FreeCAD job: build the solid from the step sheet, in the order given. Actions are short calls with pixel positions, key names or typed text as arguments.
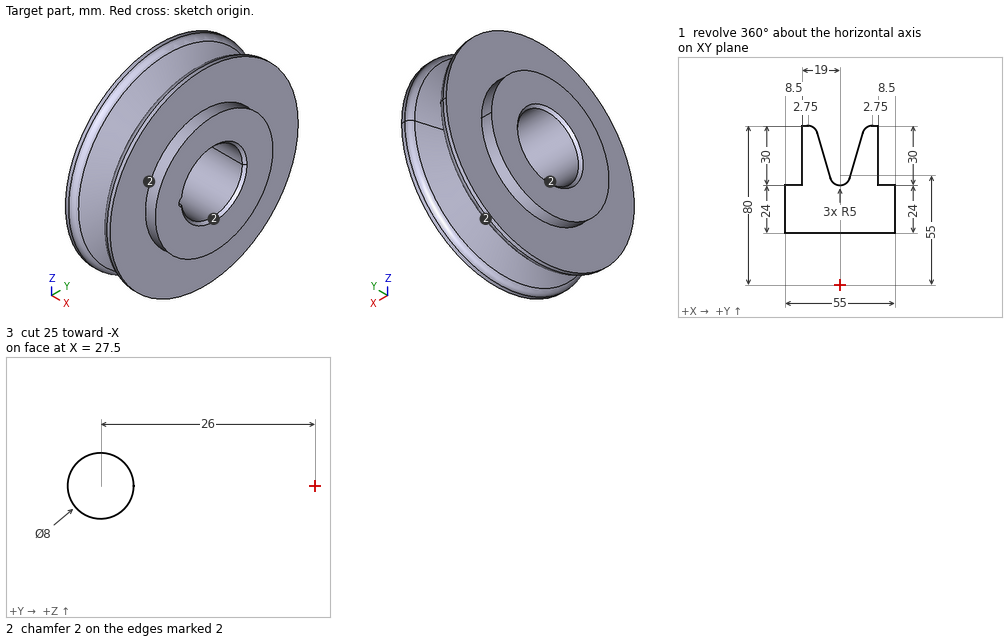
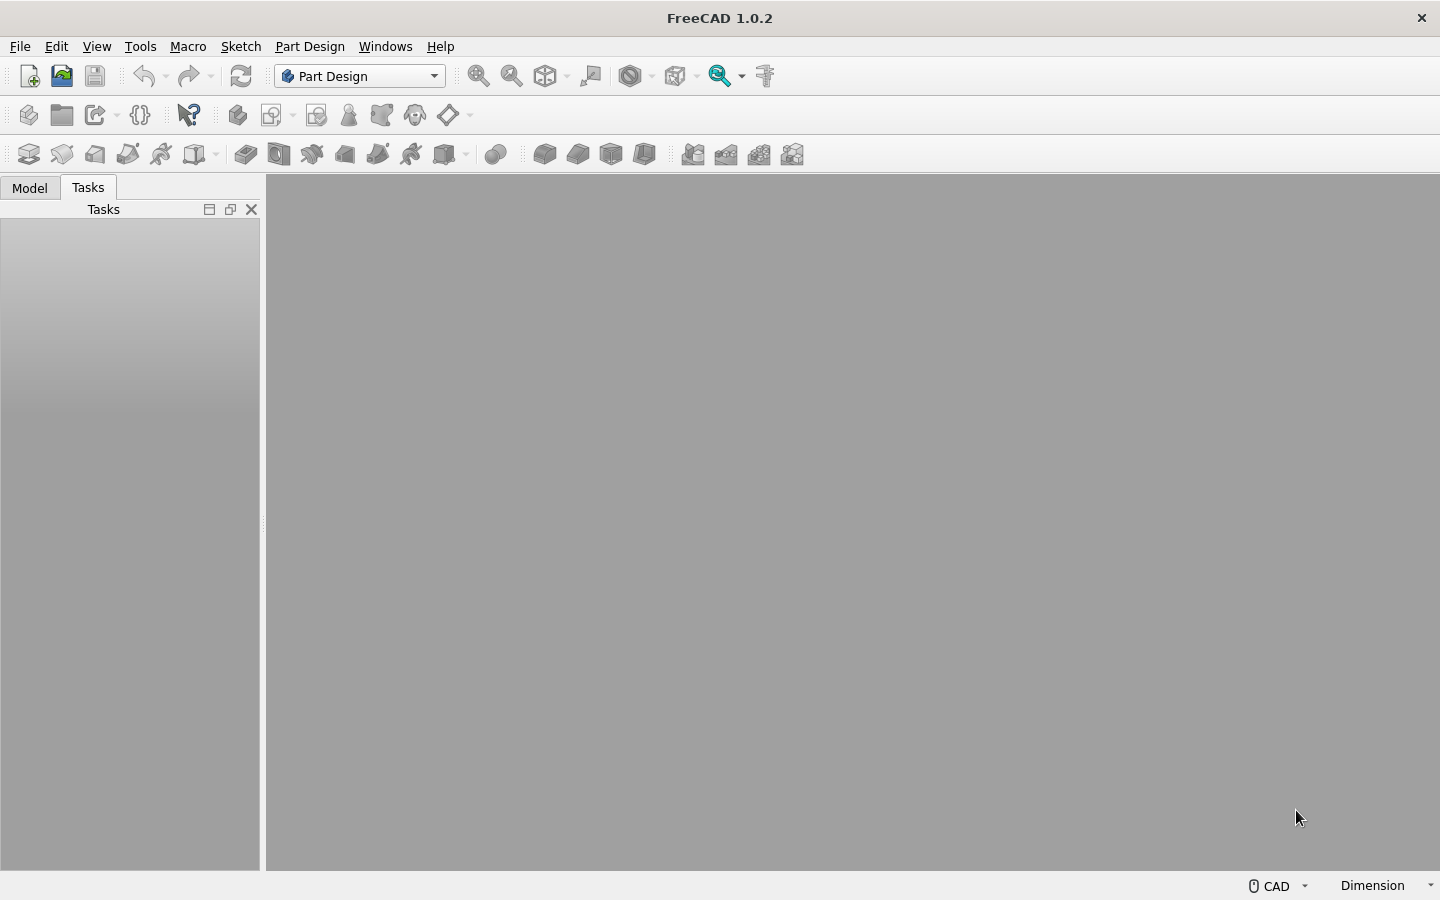
key(ctrl+n)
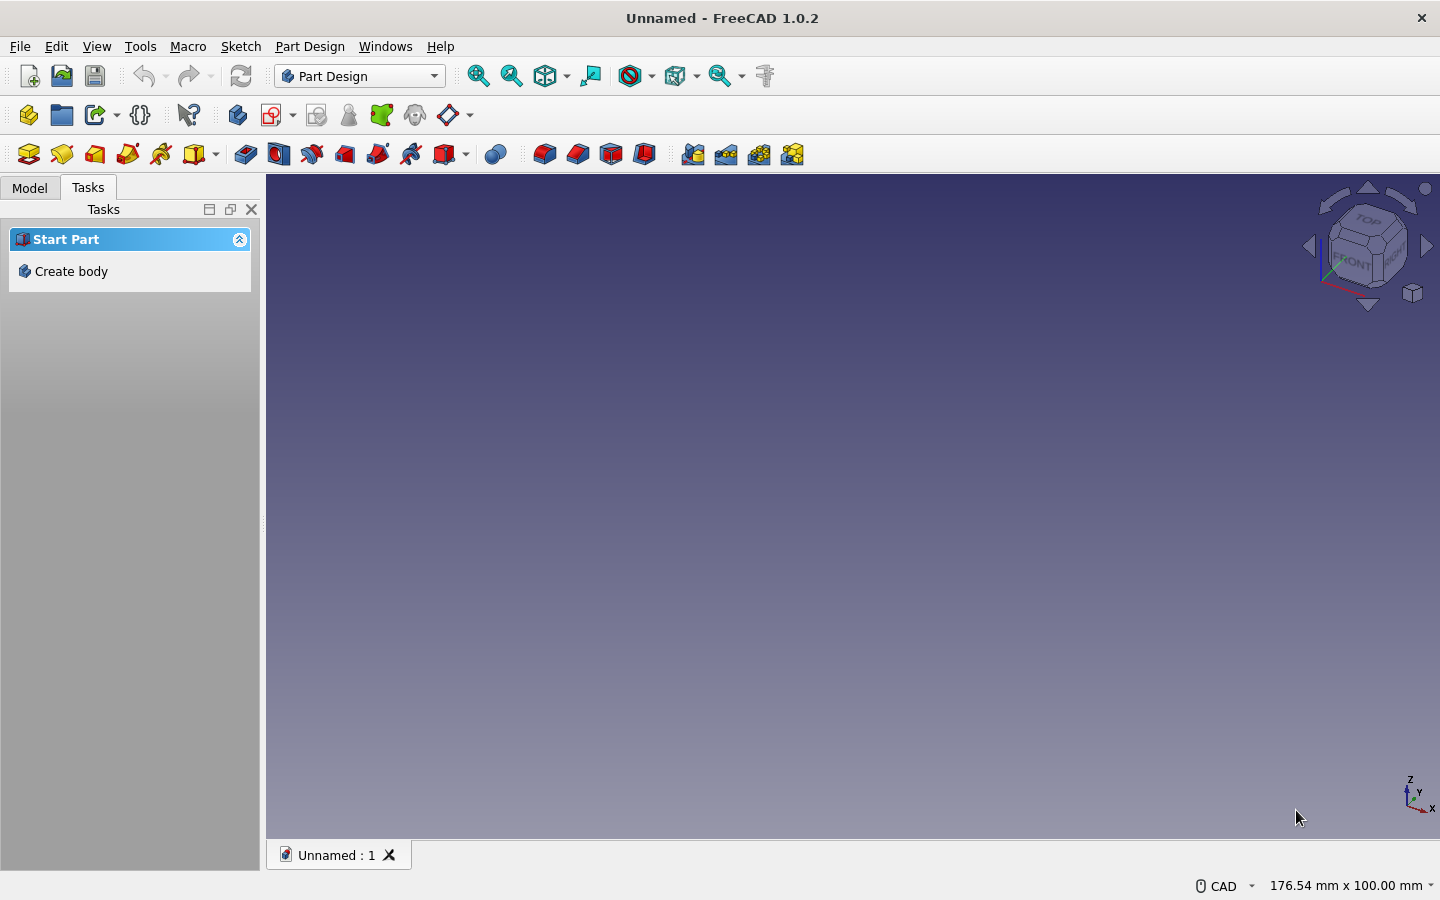
click(270, 116)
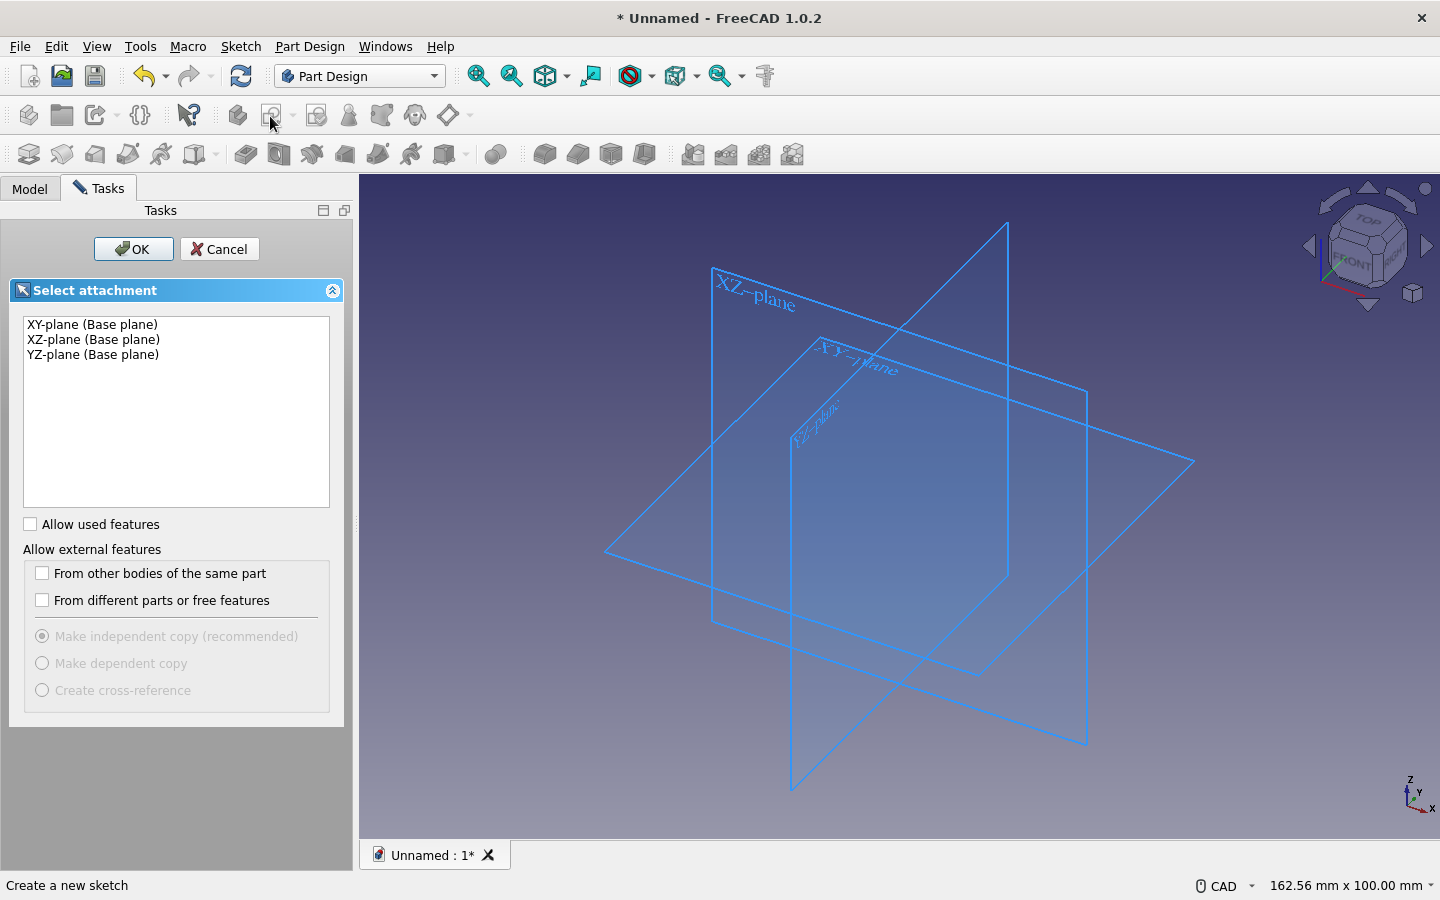
click(84, 324)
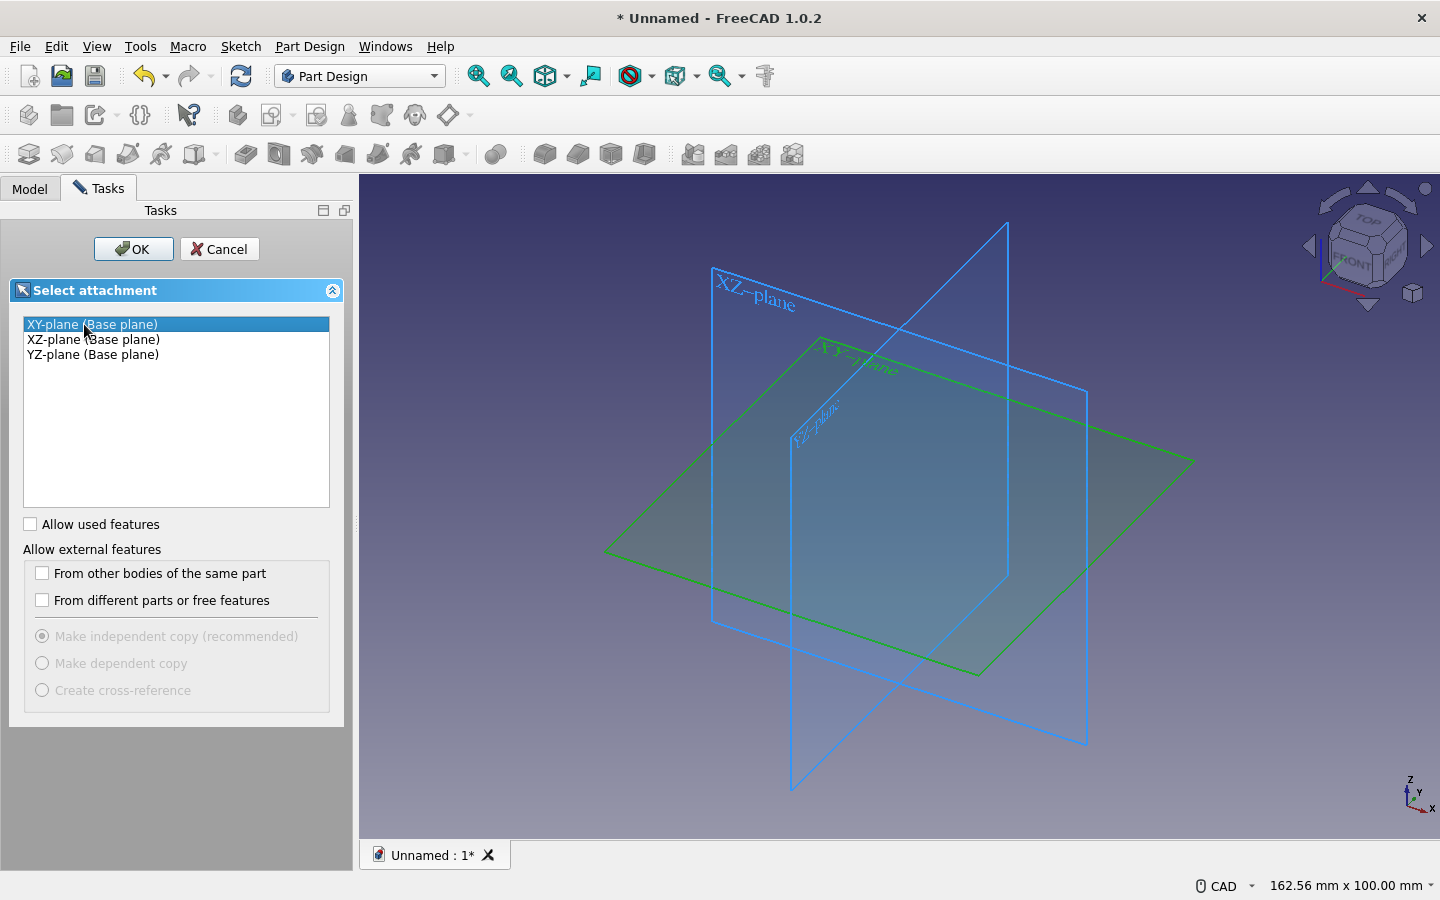
click(134, 249)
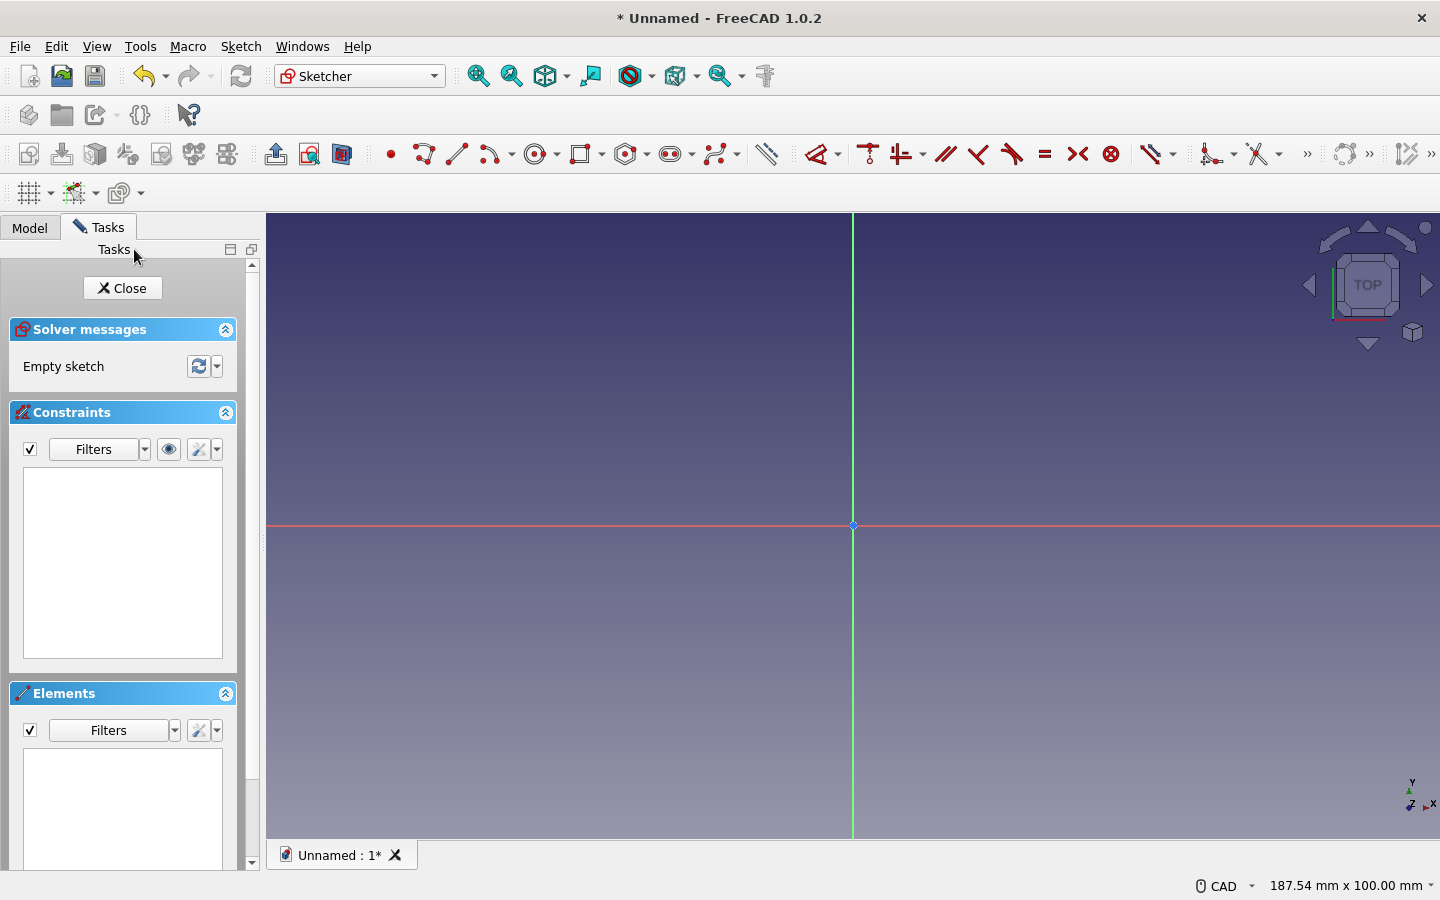
scroll(645, 811, down, 2)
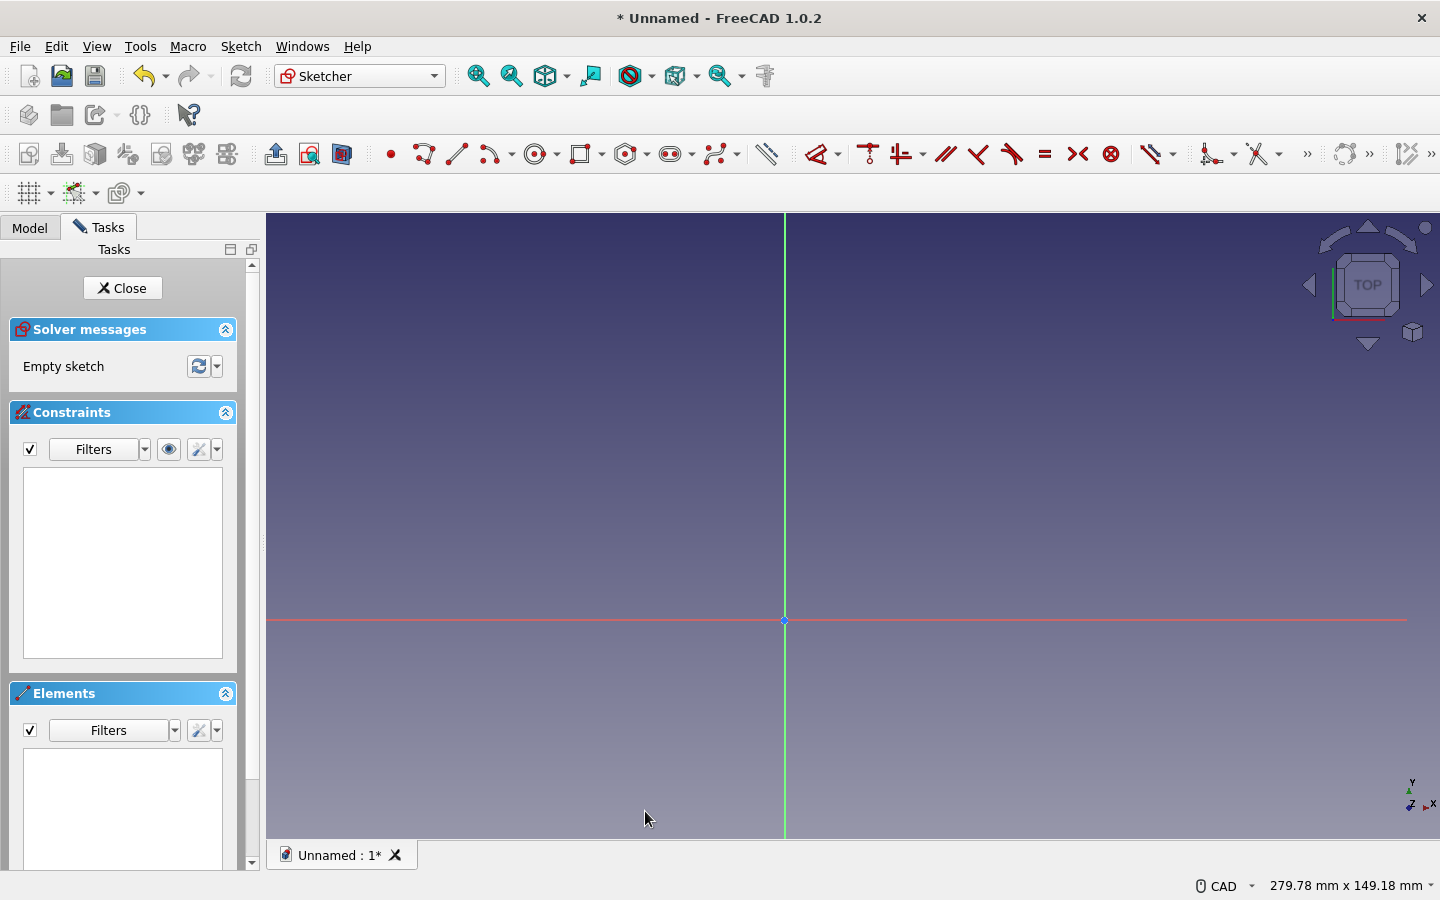
key(g)
key(l)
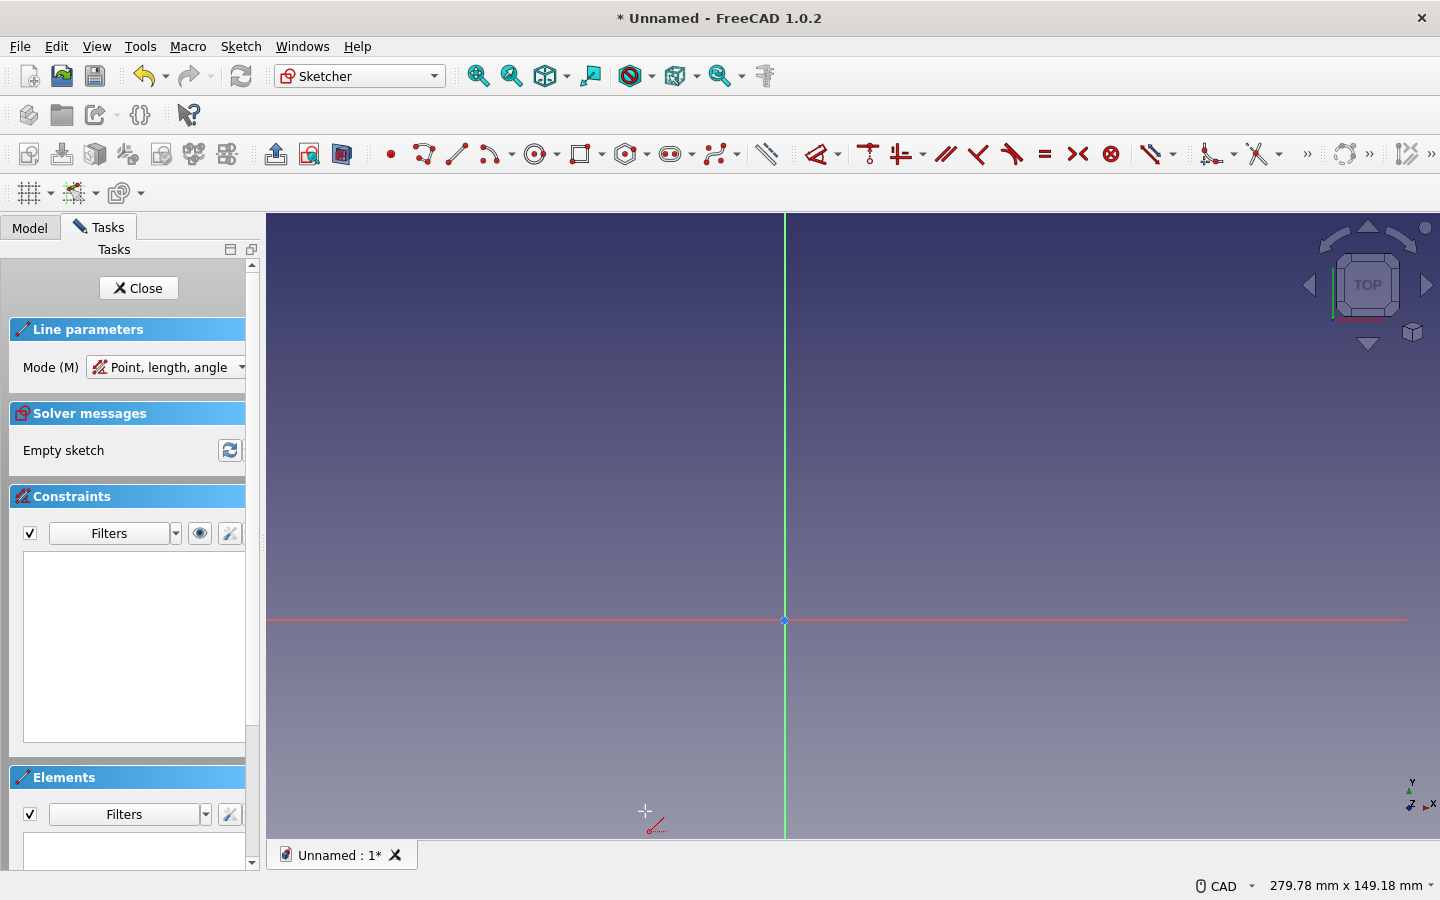
click(833, 300)
click(805, 395)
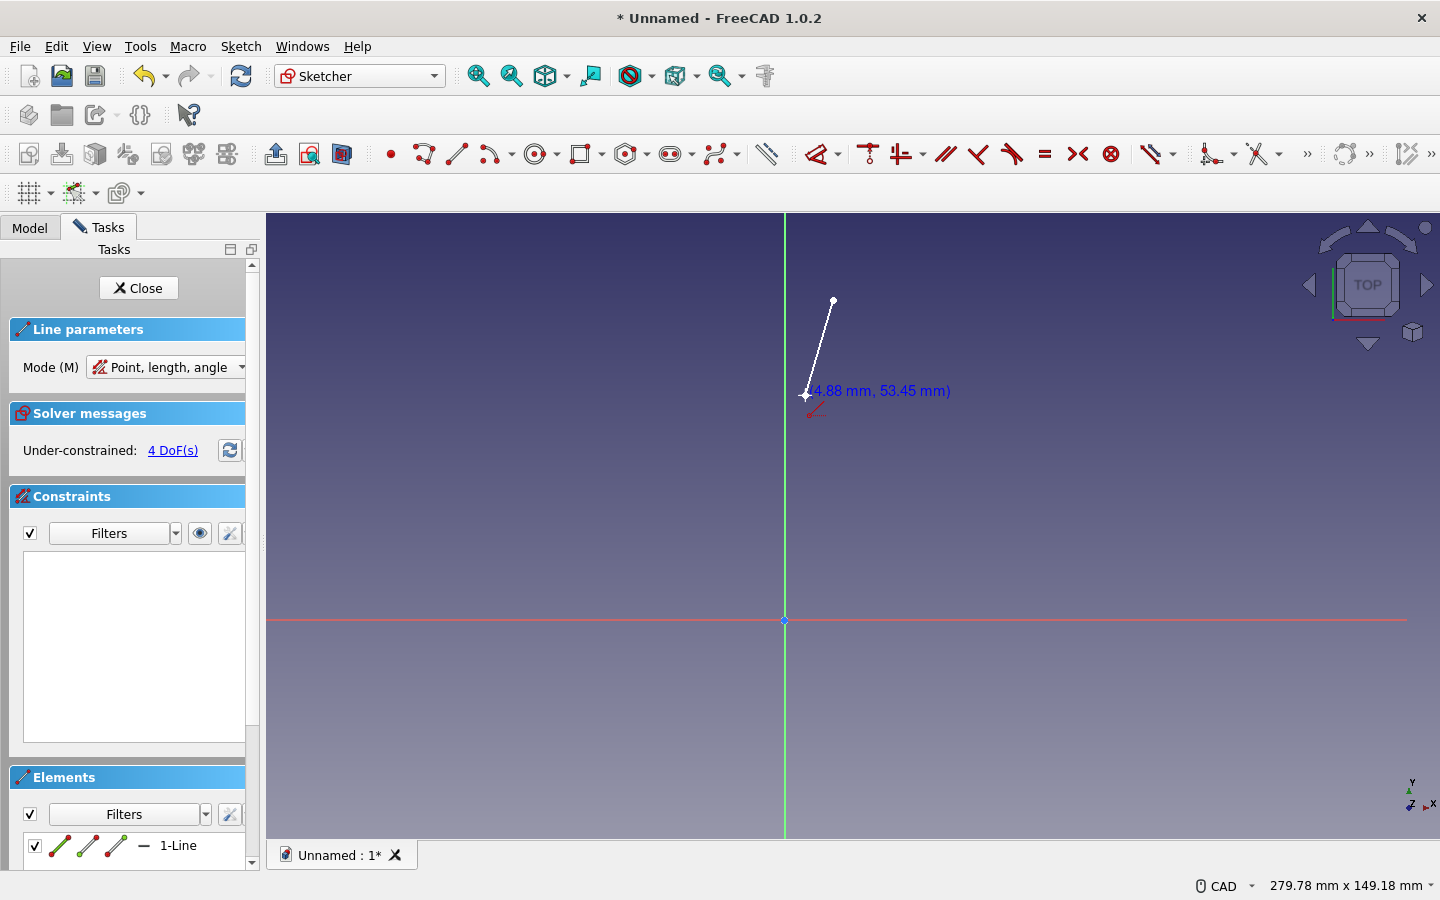
click(764, 395)
click(736, 300)